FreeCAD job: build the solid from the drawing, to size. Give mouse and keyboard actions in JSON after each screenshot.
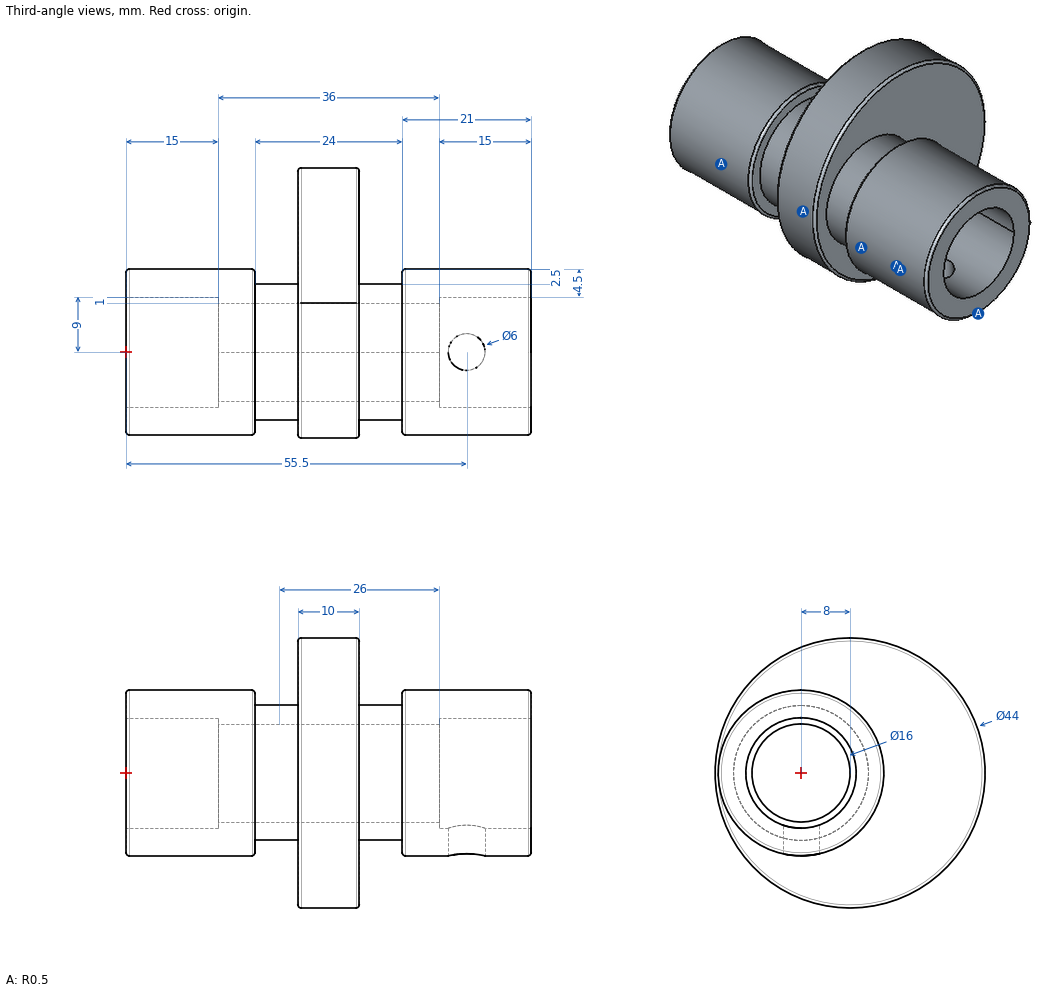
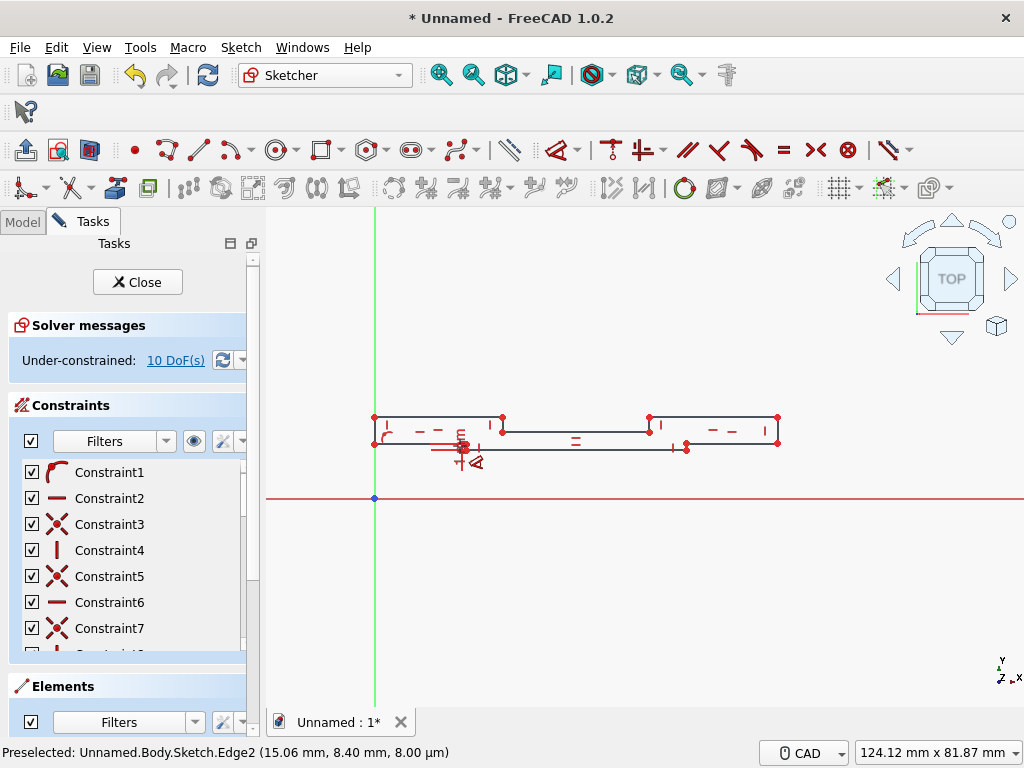
{"action": "scroll", "coordinate": [686, 448], "scroll_direction": "up", "scroll_amount": 10}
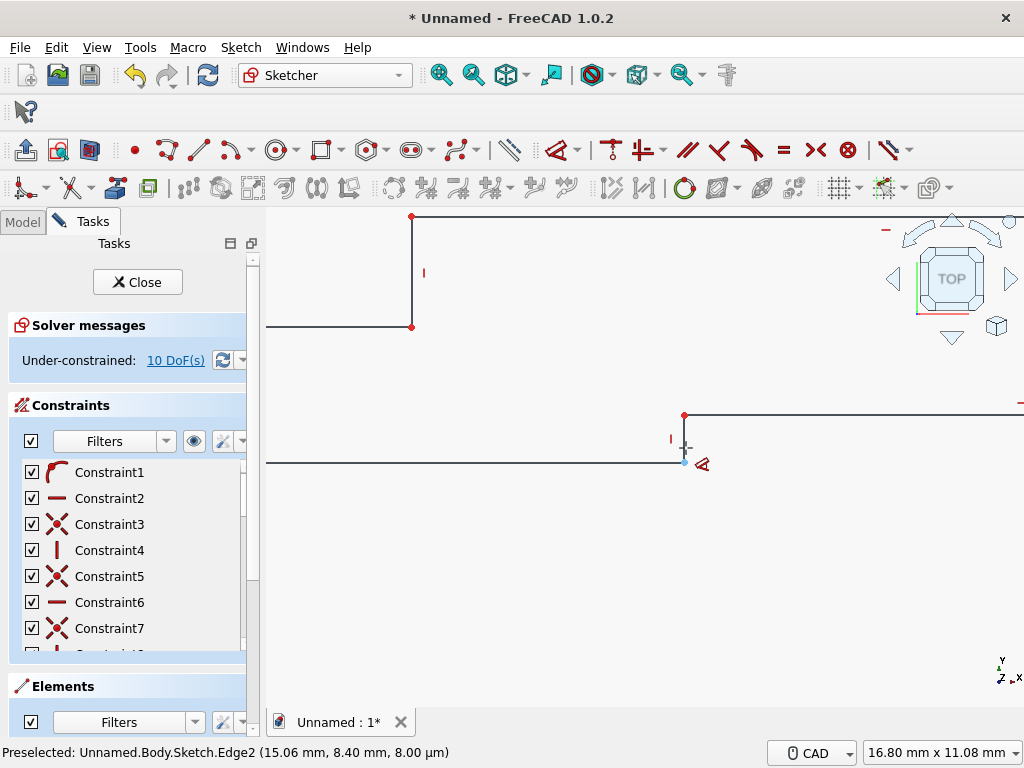
{"action": "left_click", "coordinate": [684, 448]}
{"action": "left_click", "coordinate": [718, 439]}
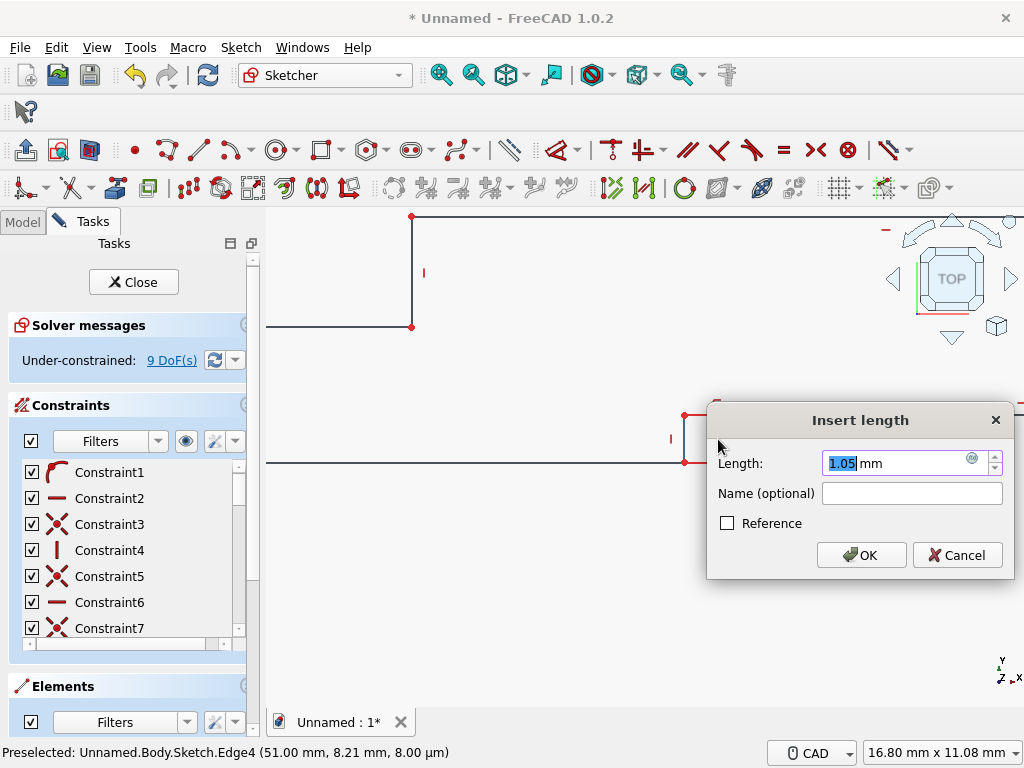
{"action": "type", "text": "1"}
{"action": "key", "text": "Return"}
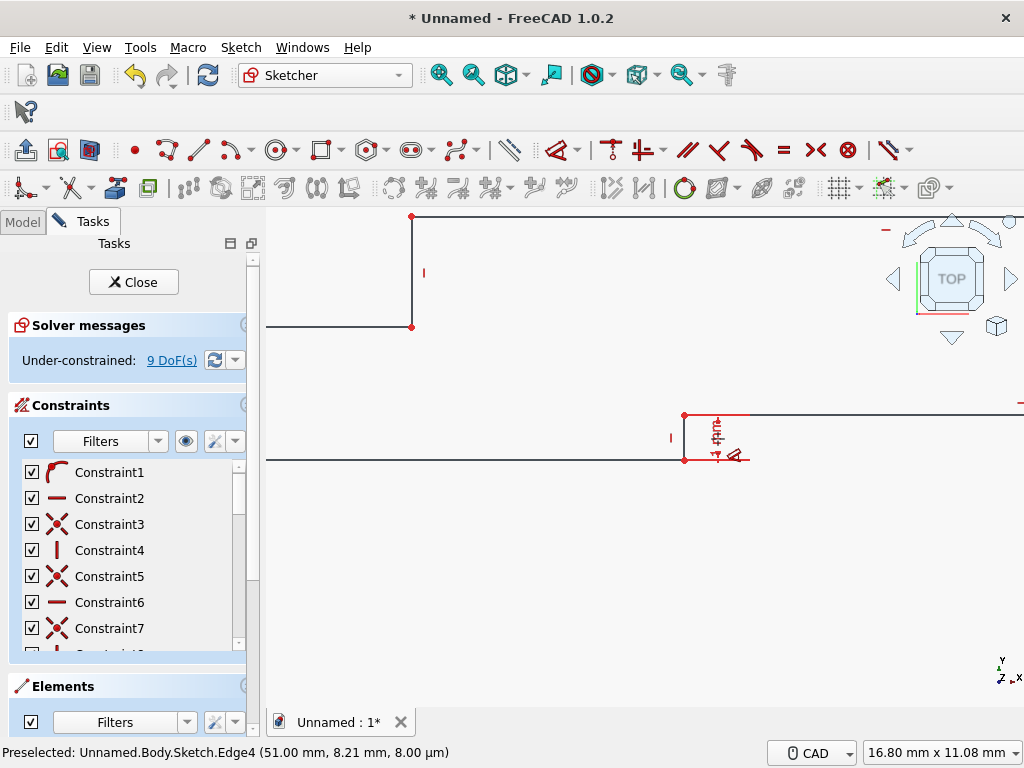
{"action": "scroll", "coordinate": [687, 448], "scroll_direction": "down", "scroll_amount": 10}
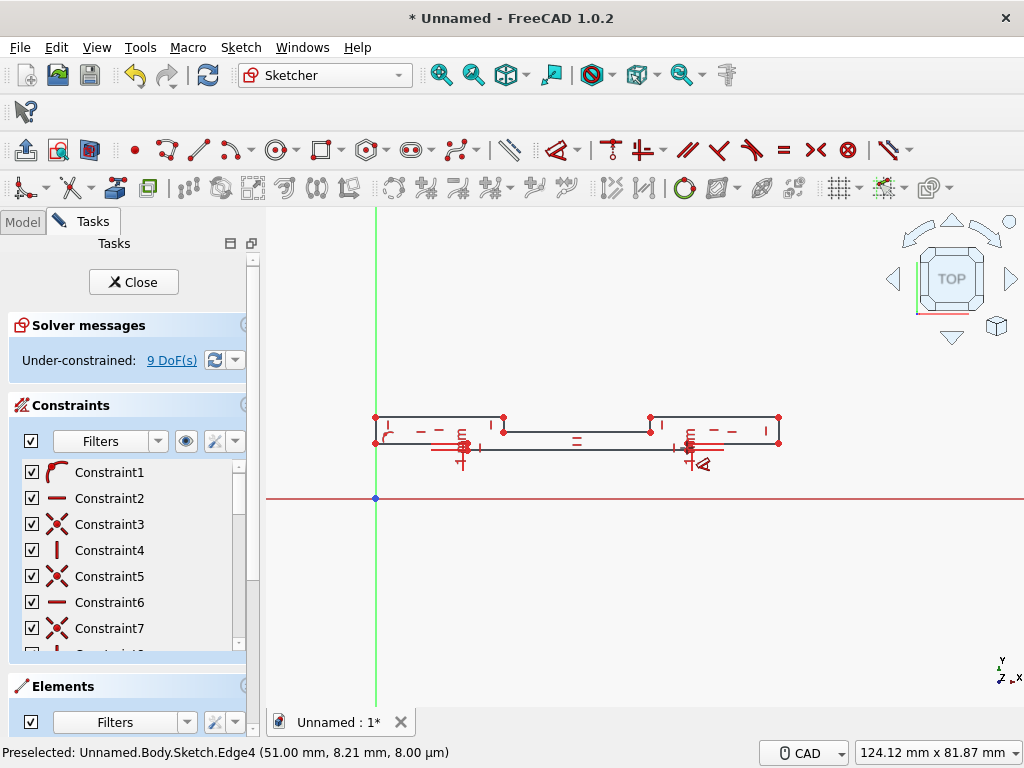
{"action": "left_click", "coordinate": [403, 444]}
{"action": "left_click", "coordinate": [422, 478]}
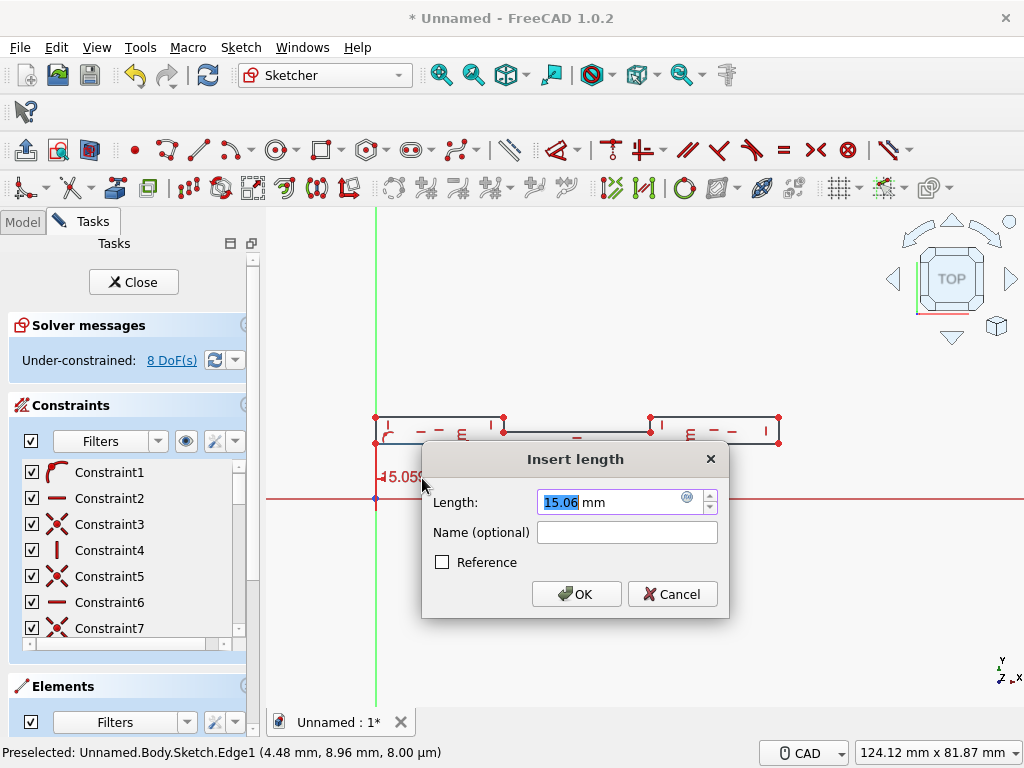
{"action": "type", "text": "15"}
{"action": "key", "text": "Return"}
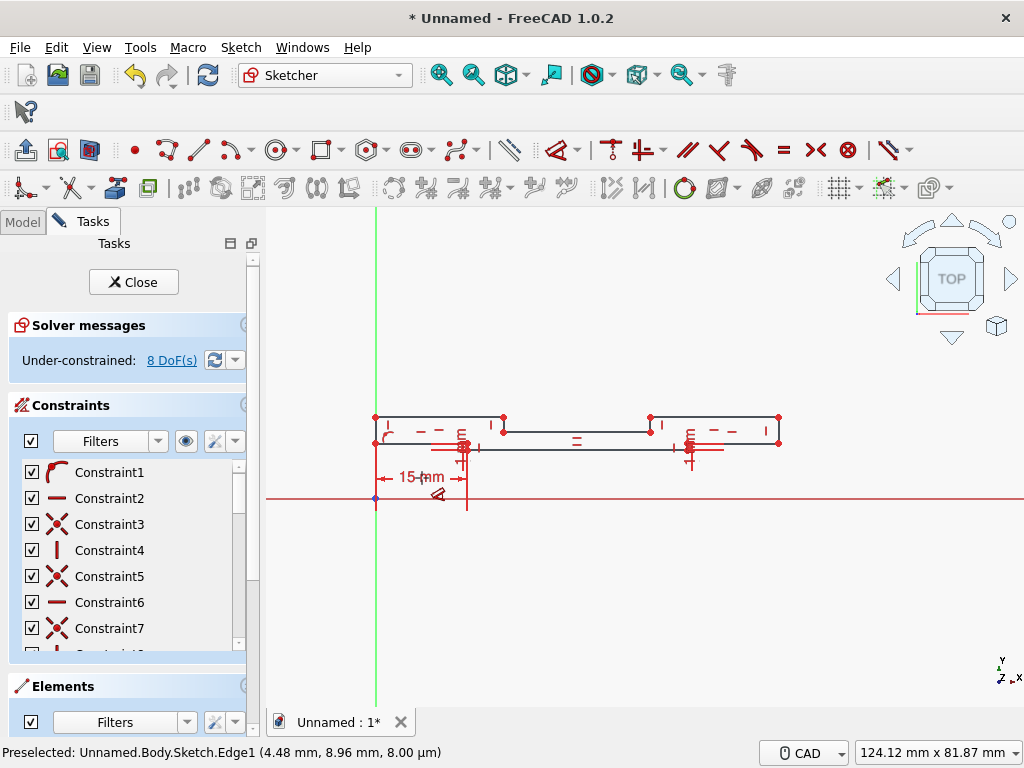
{"action": "left_click", "coordinate": [533, 450]}
{"action": "left_click", "coordinate": [577, 416]}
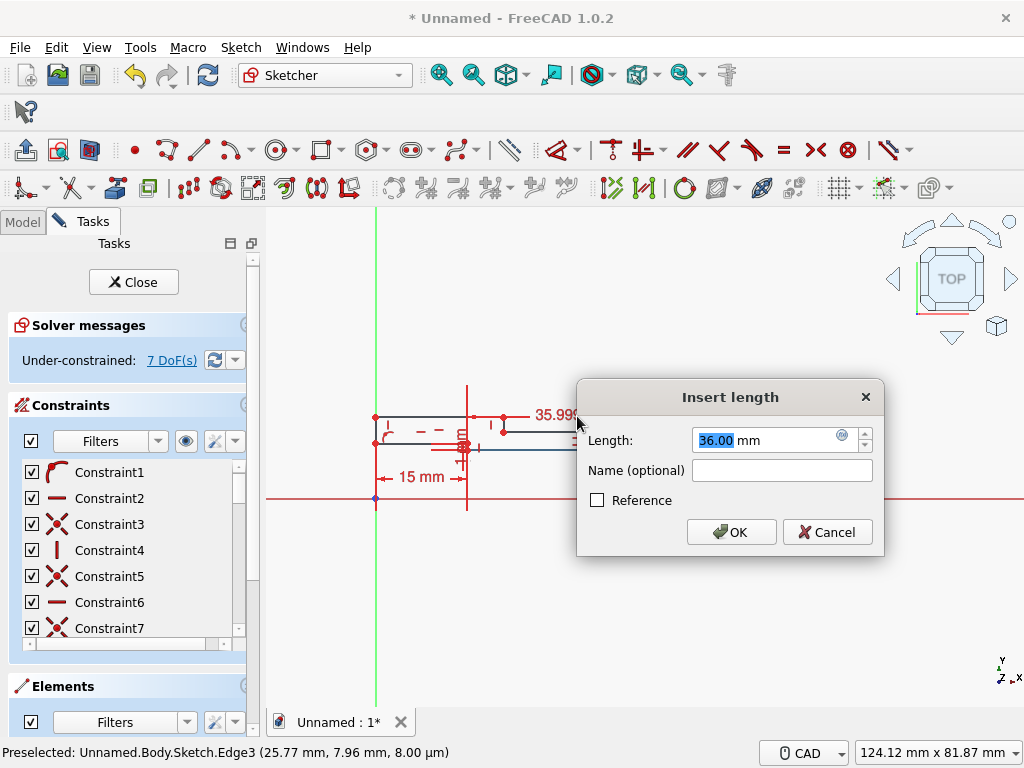
{"action": "type", "text": "36"}
{"action": "key", "text": "Return"}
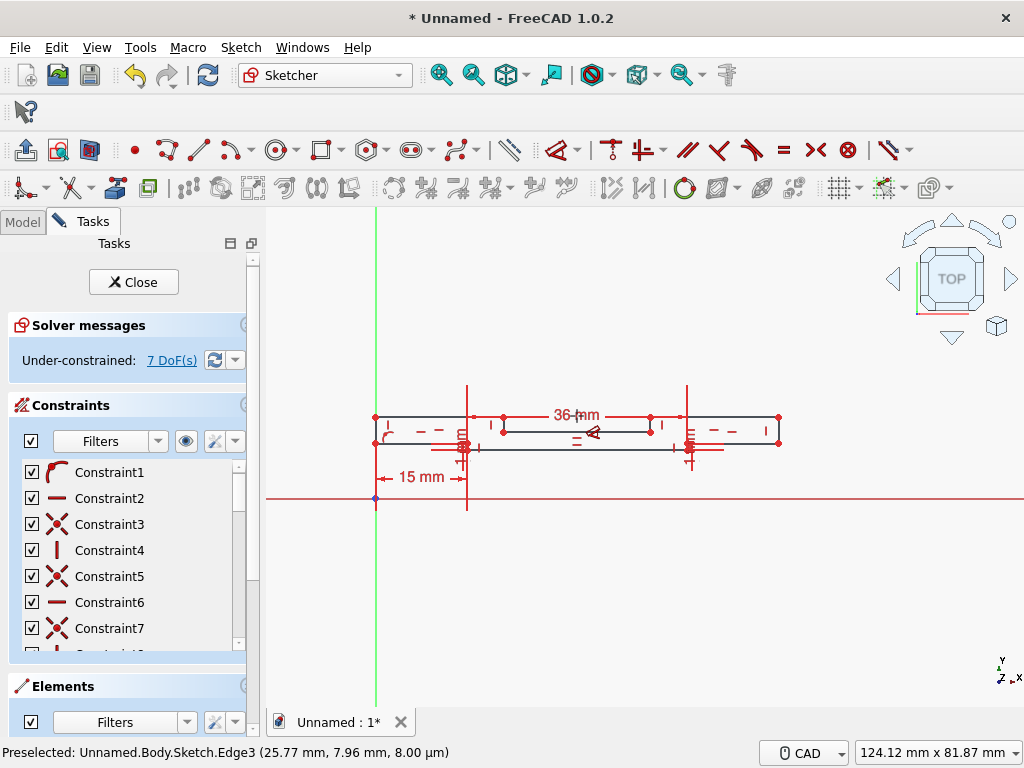
{"action": "left_click", "coordinate": [715, 444]}
{"action": "left_click", "coordinate": [733, 478]}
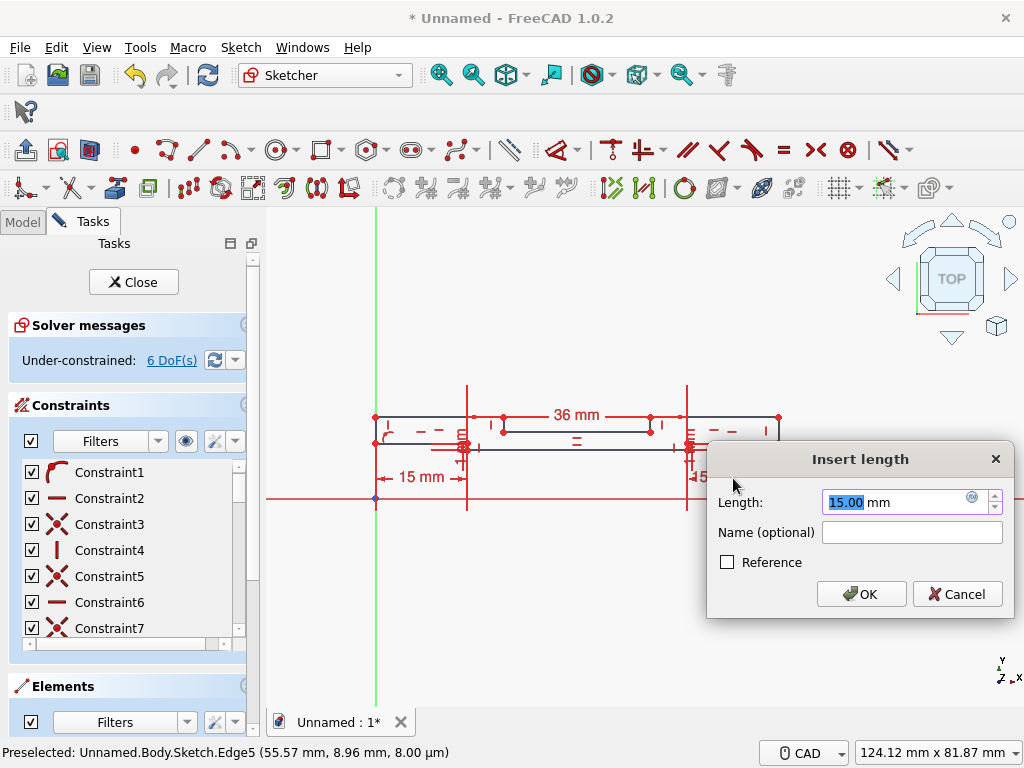
{"action": "type", "text": "15"}
{"action": "key", "text": "Return"}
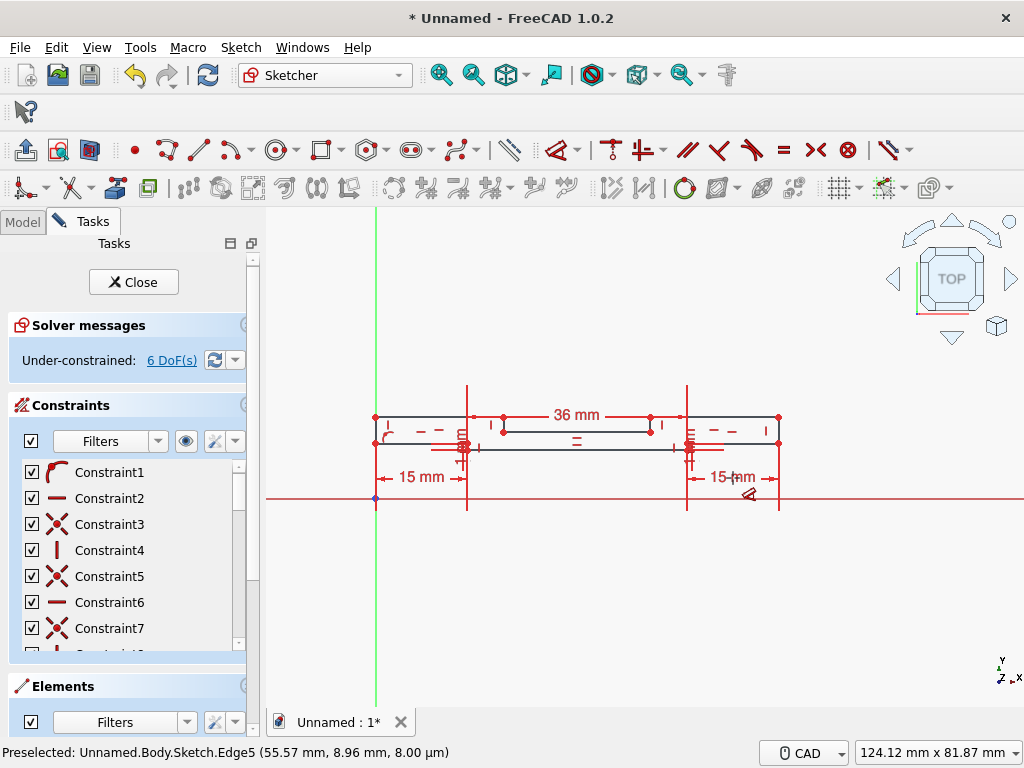
{"action": "left_click", "coordinate": [740, 417]}
{"action": "left_click", "coordinate": [714, 383]}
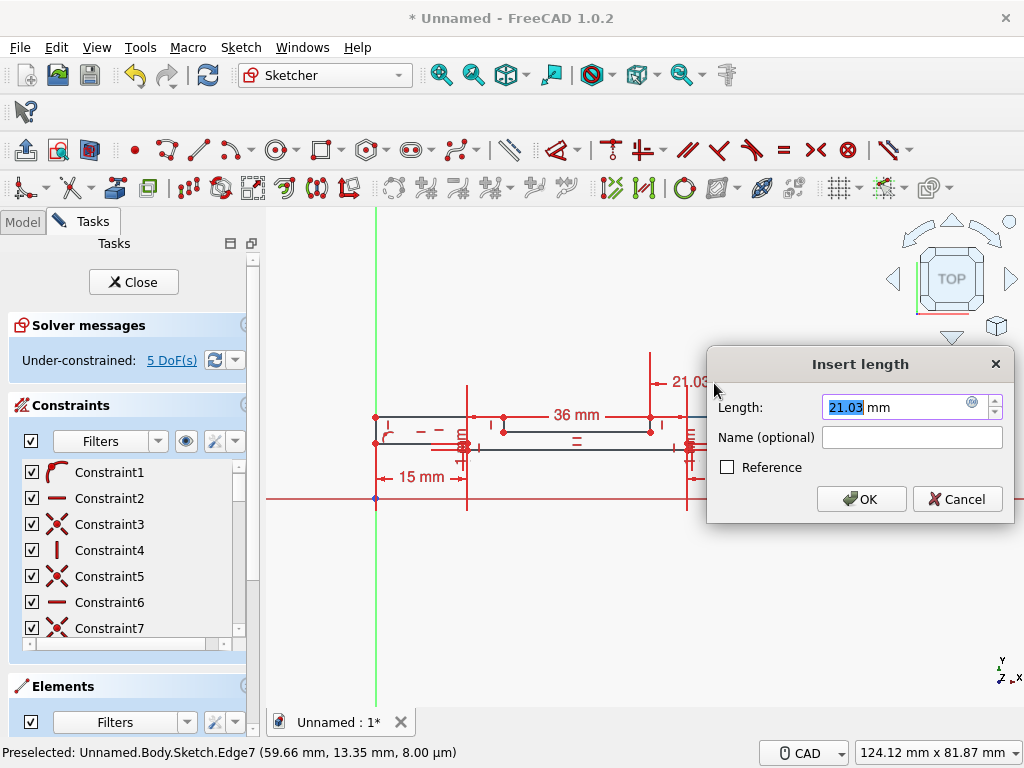
{"action": "type", "text": "21"}
{"action": "key", "text": "Return"}